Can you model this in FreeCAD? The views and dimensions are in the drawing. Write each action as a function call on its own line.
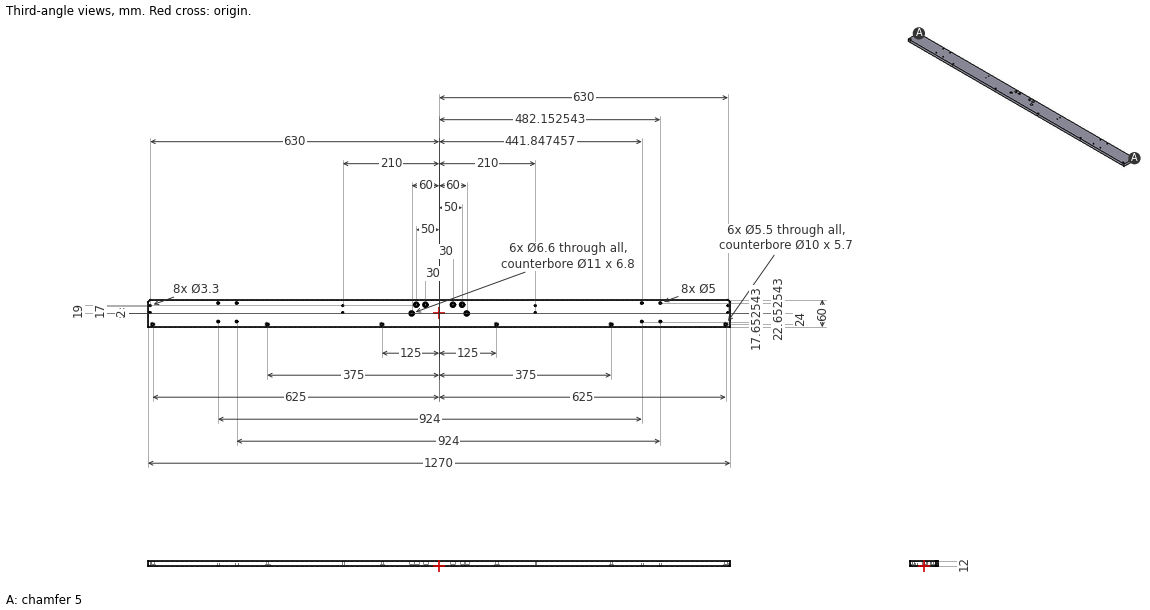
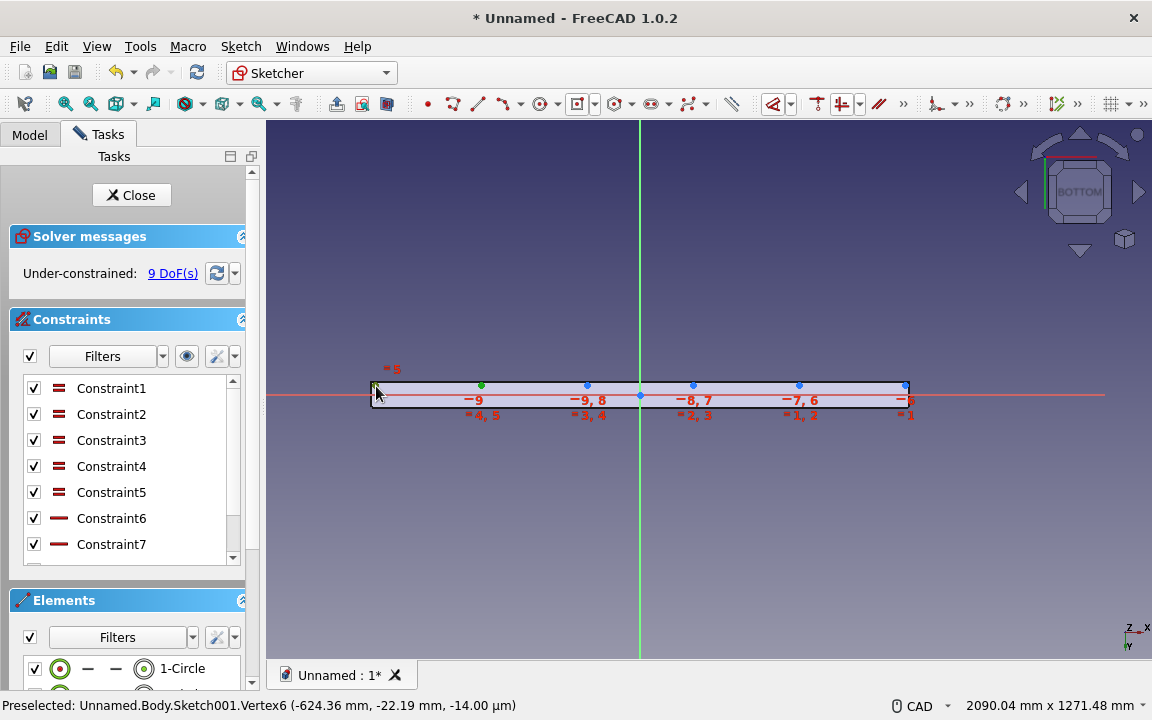
key(h)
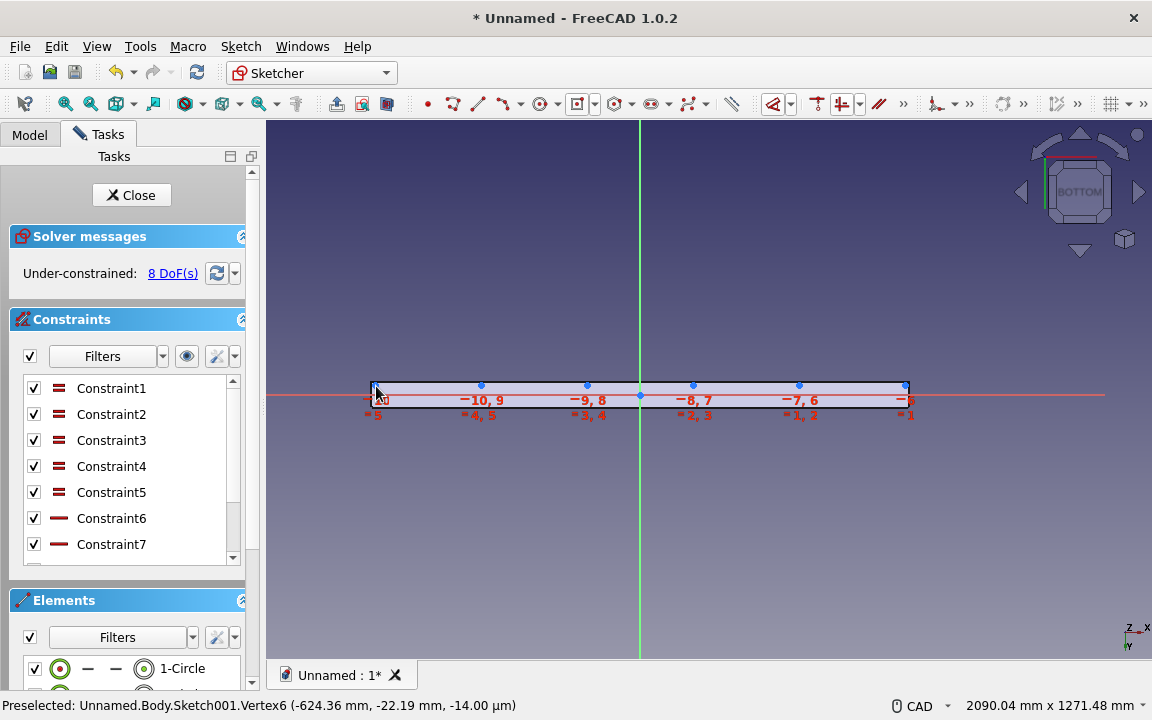
scroll(904, 385, up, 15)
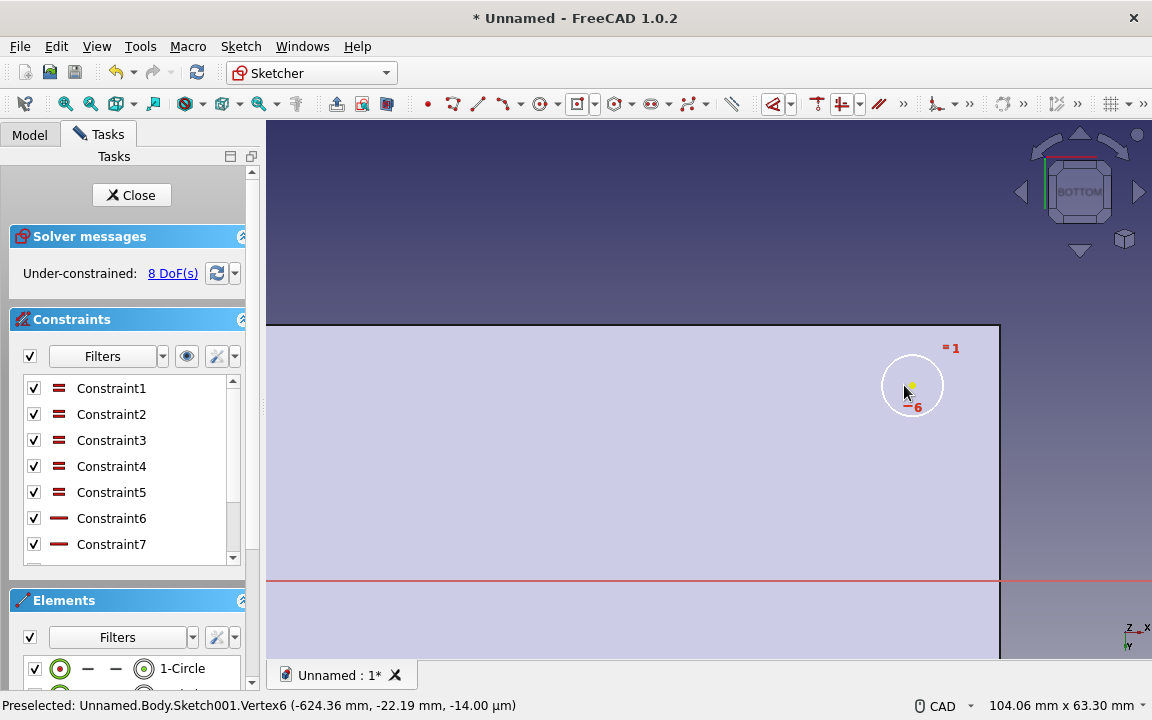
click(882, 385)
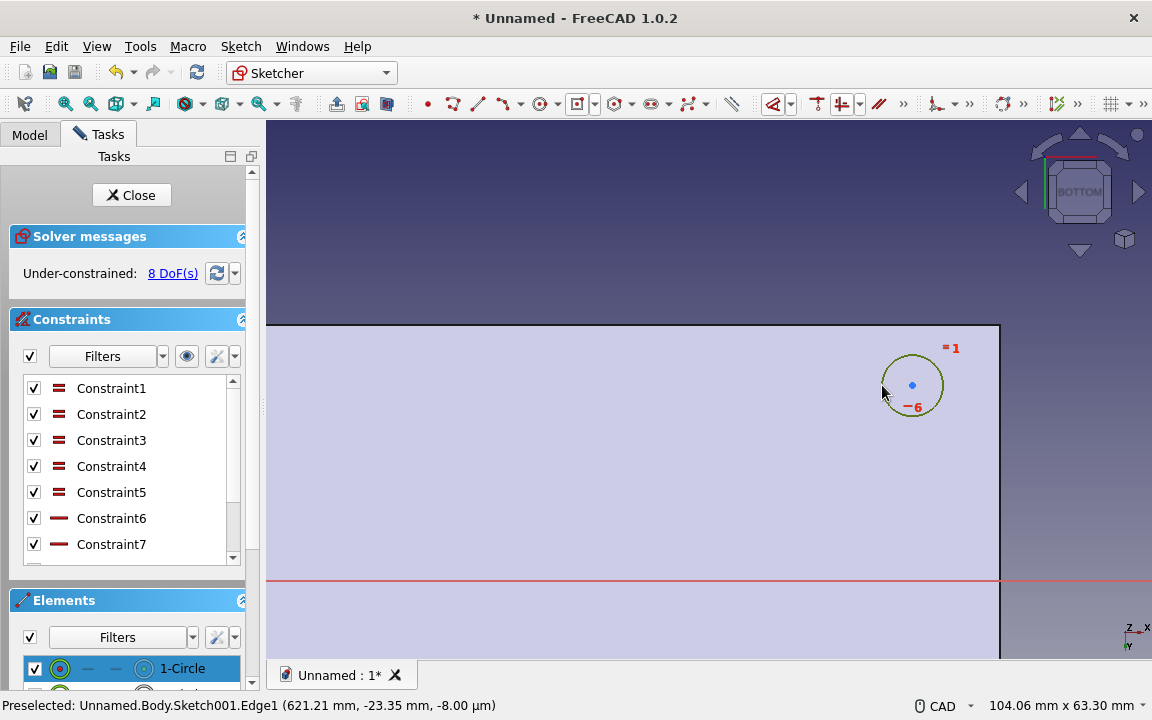
click(790, 104)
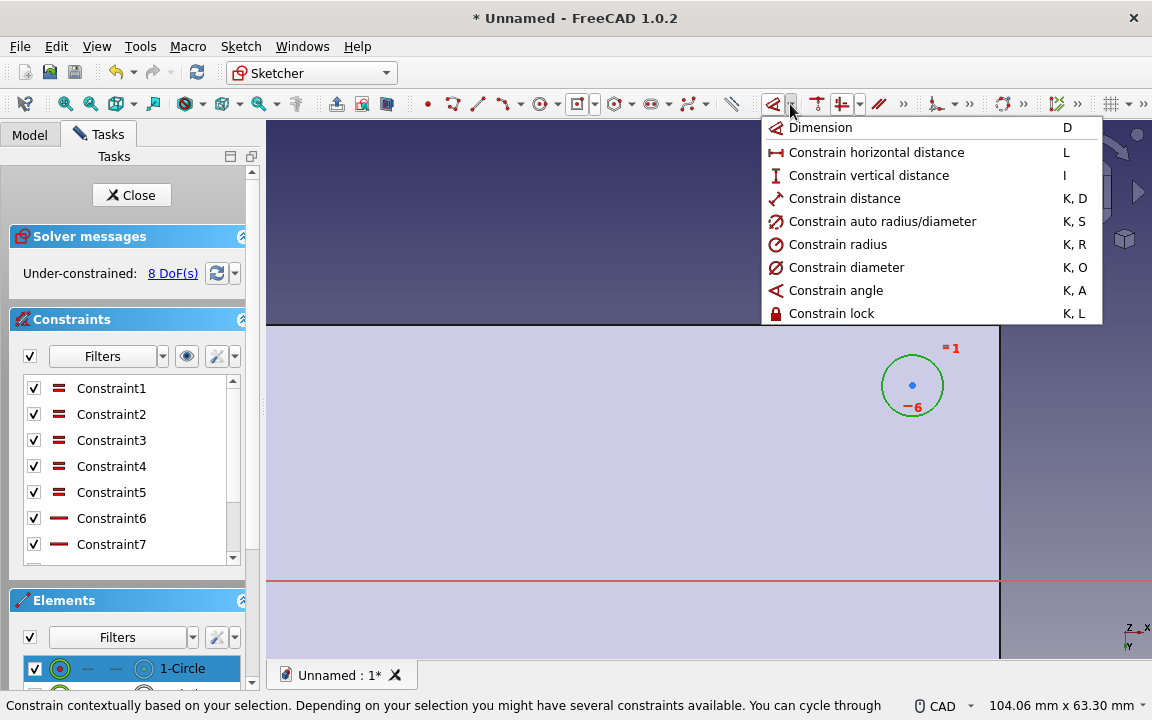
click(932, 268)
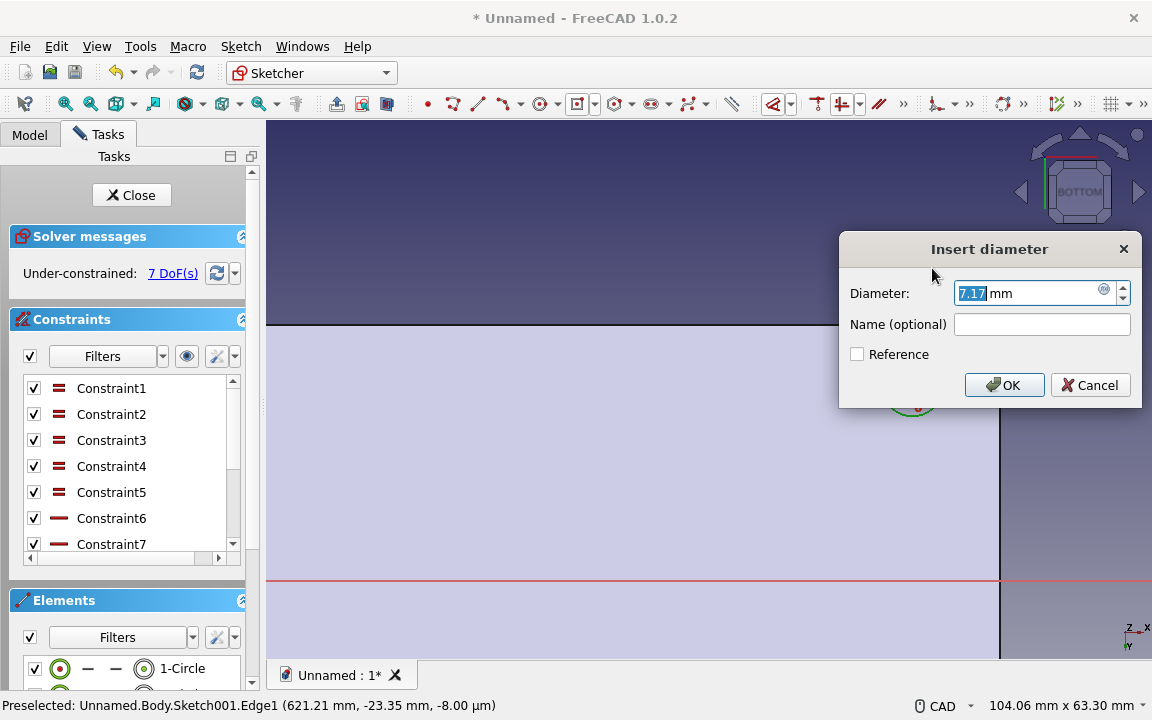
text(5.5)
key(Return)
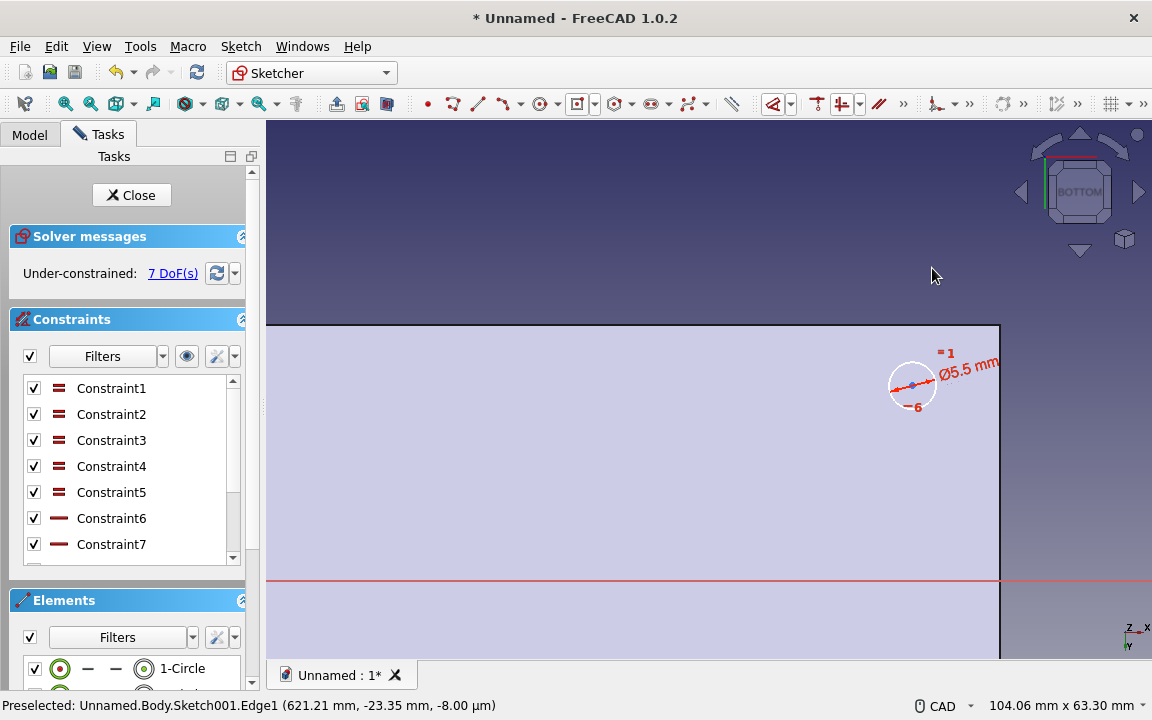
scroll(905, 385, down, 15)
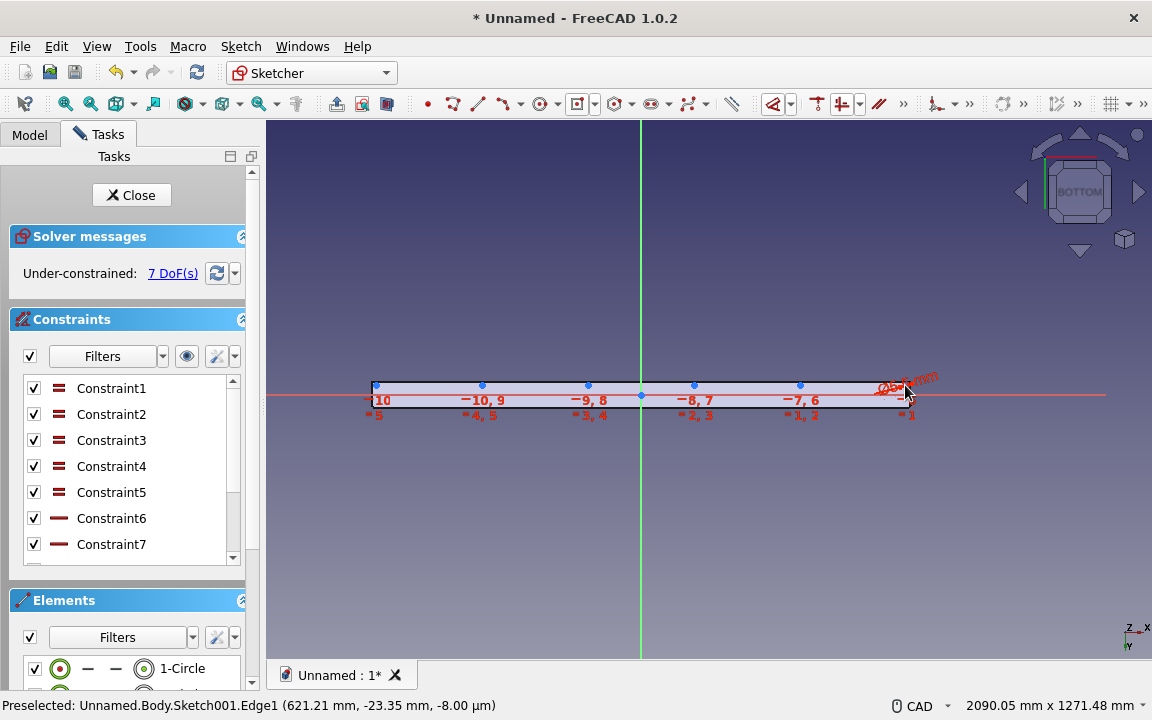
scroll(906, 386, up, 7)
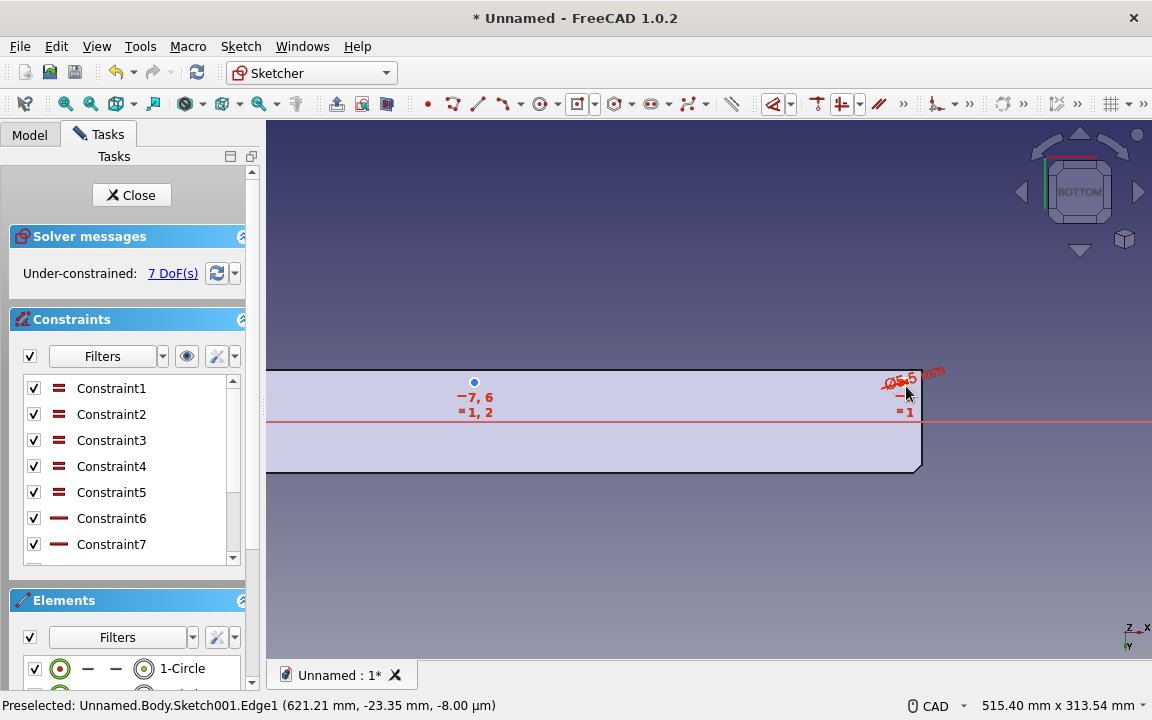
click(904, 382)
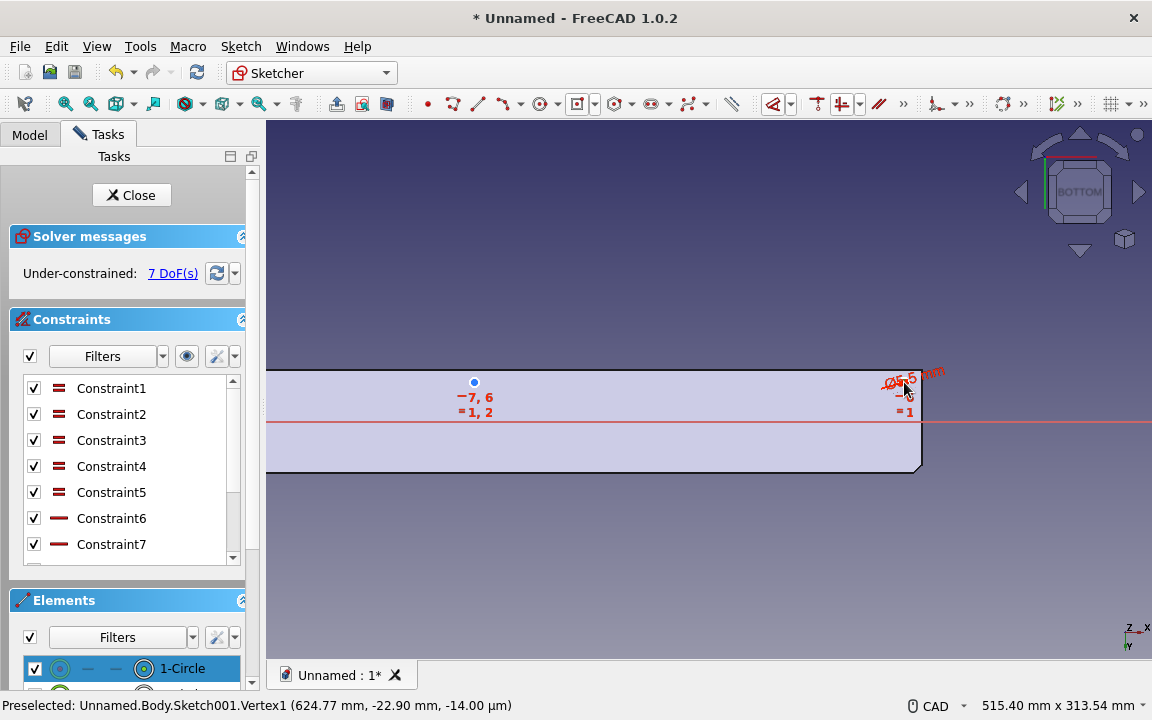
key(i)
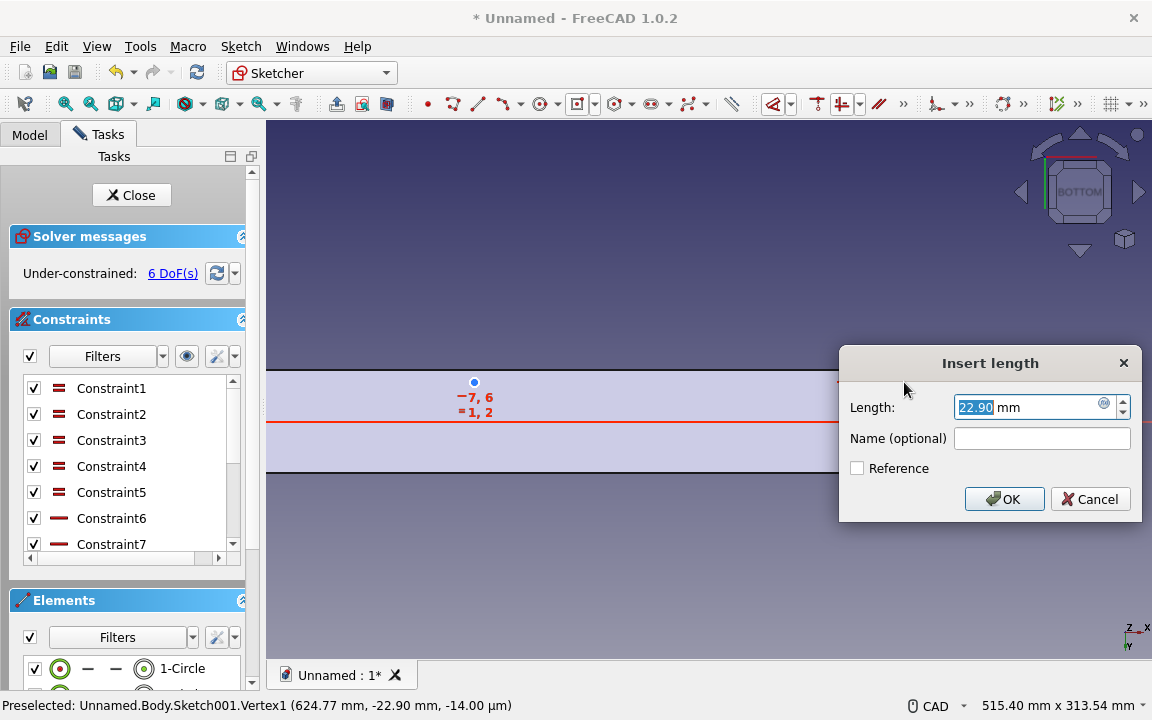
text(24)
key(Return)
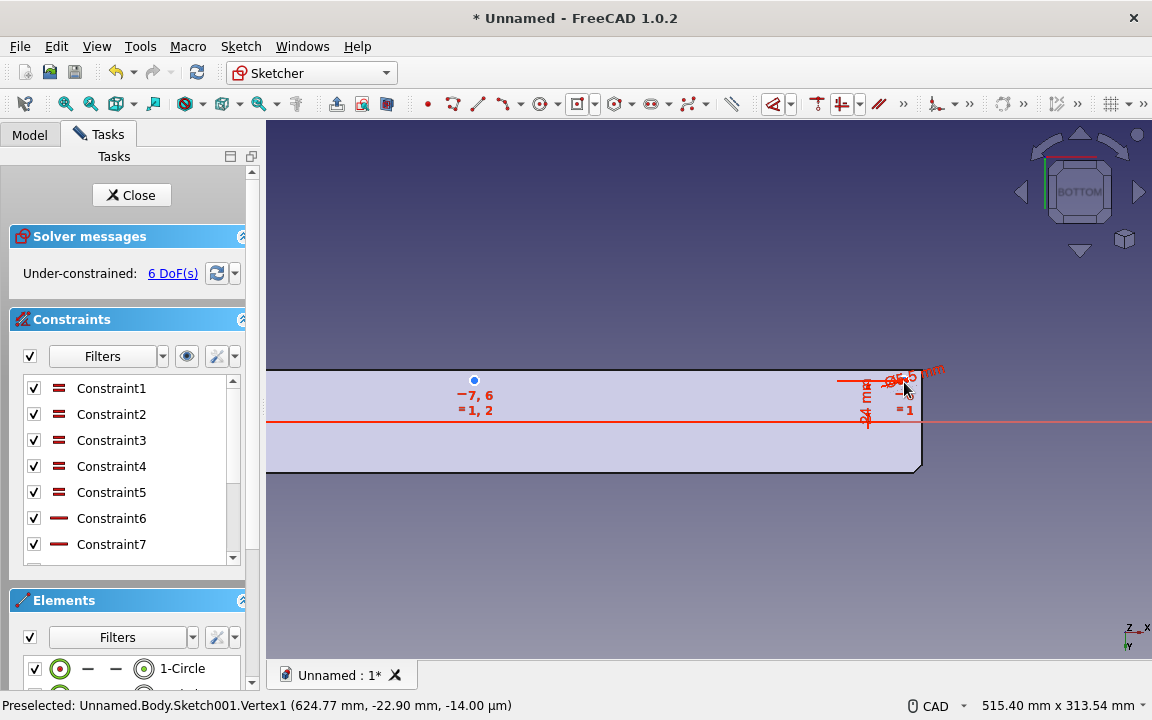
scroll(906, 386, down, 7)